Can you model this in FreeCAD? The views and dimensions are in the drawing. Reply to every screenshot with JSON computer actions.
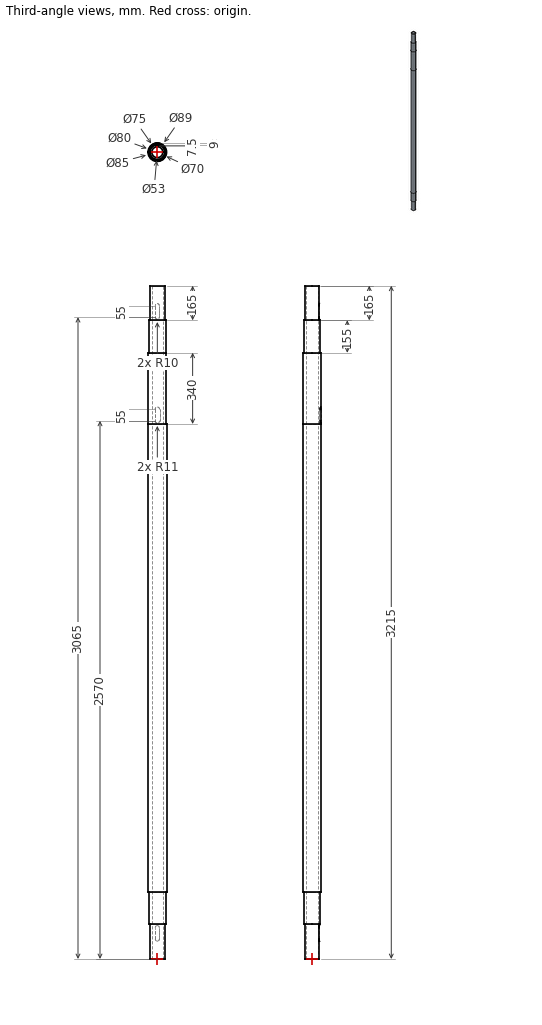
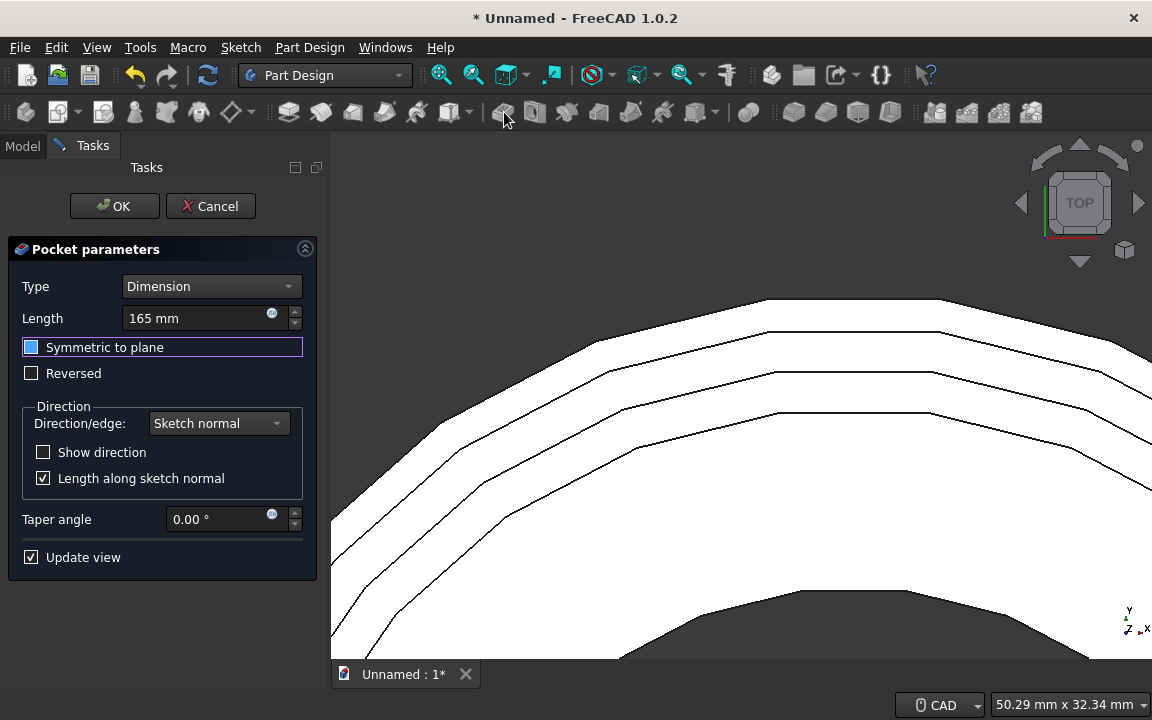
{"action": "left_click", "coordinate": [30, 373]}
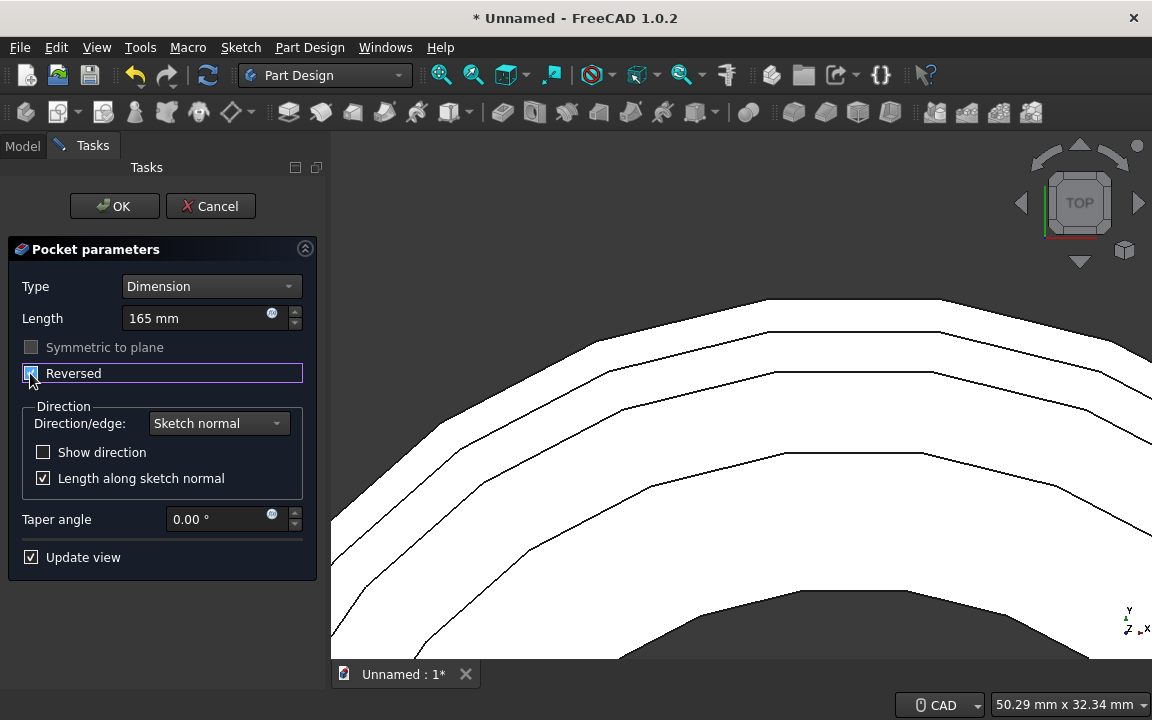
{"action": "left_click", "coordinate": [115, 206]}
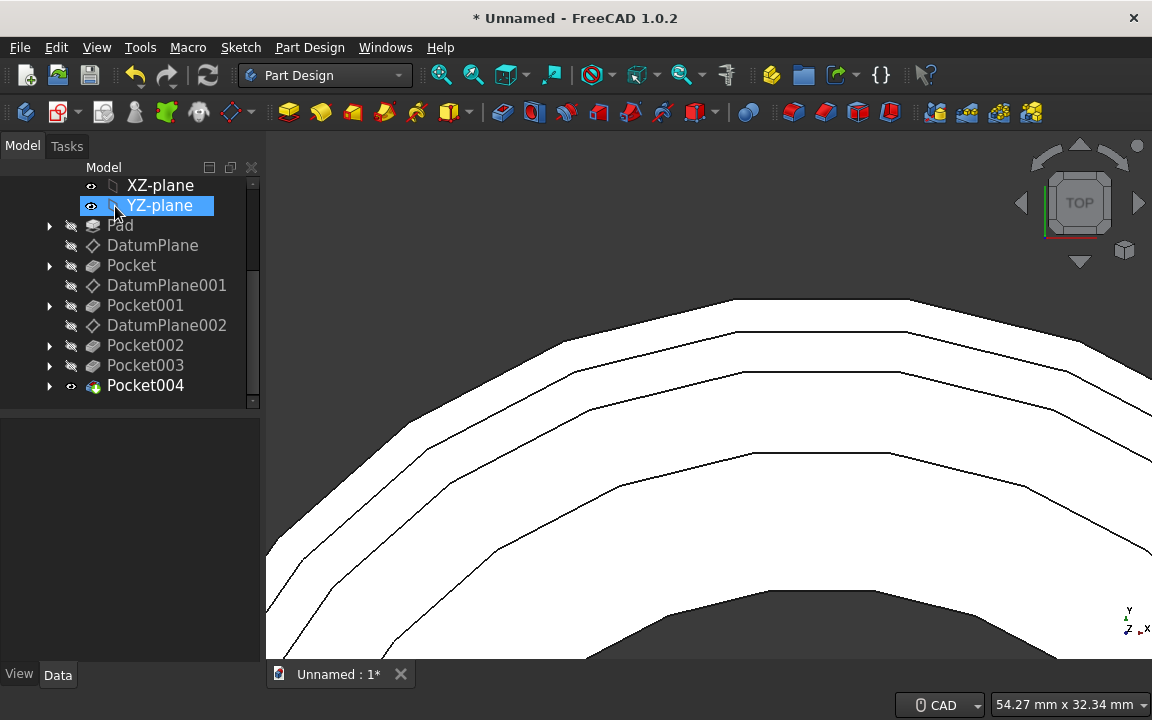
{"action": "left_click", "coordinate": [442, 76]}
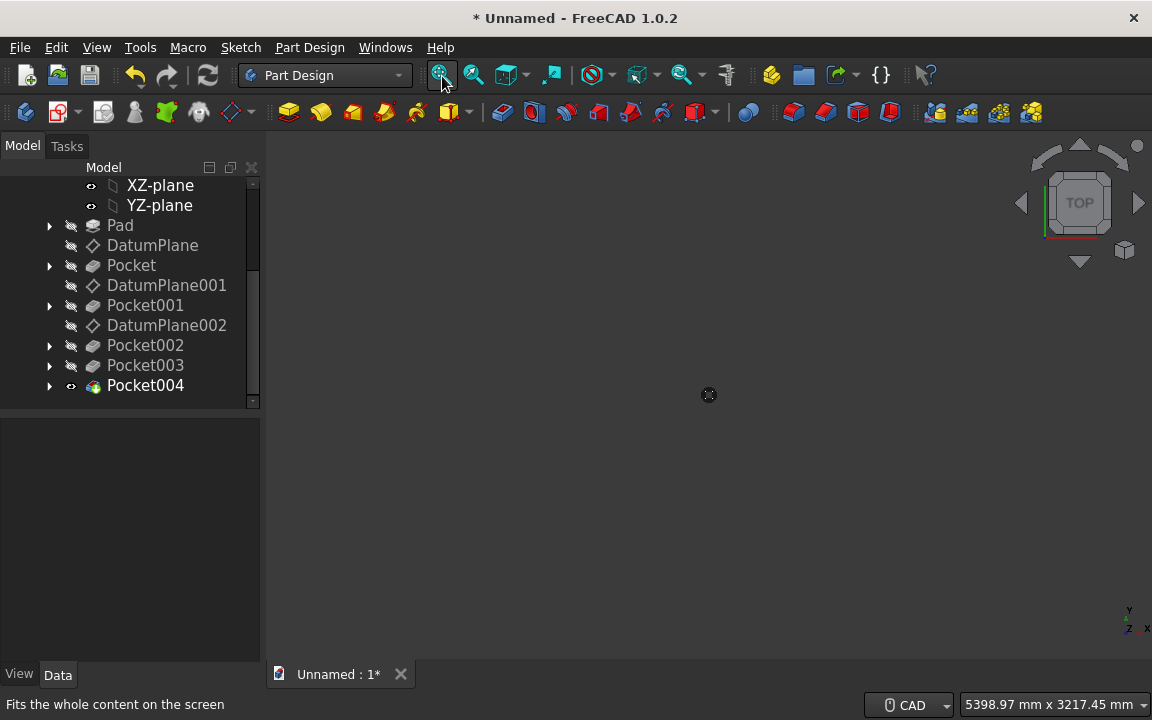
{"action": "scroll", "coordinate": [160, 281], "scroll_direction": "down", "scroll_amount": 3}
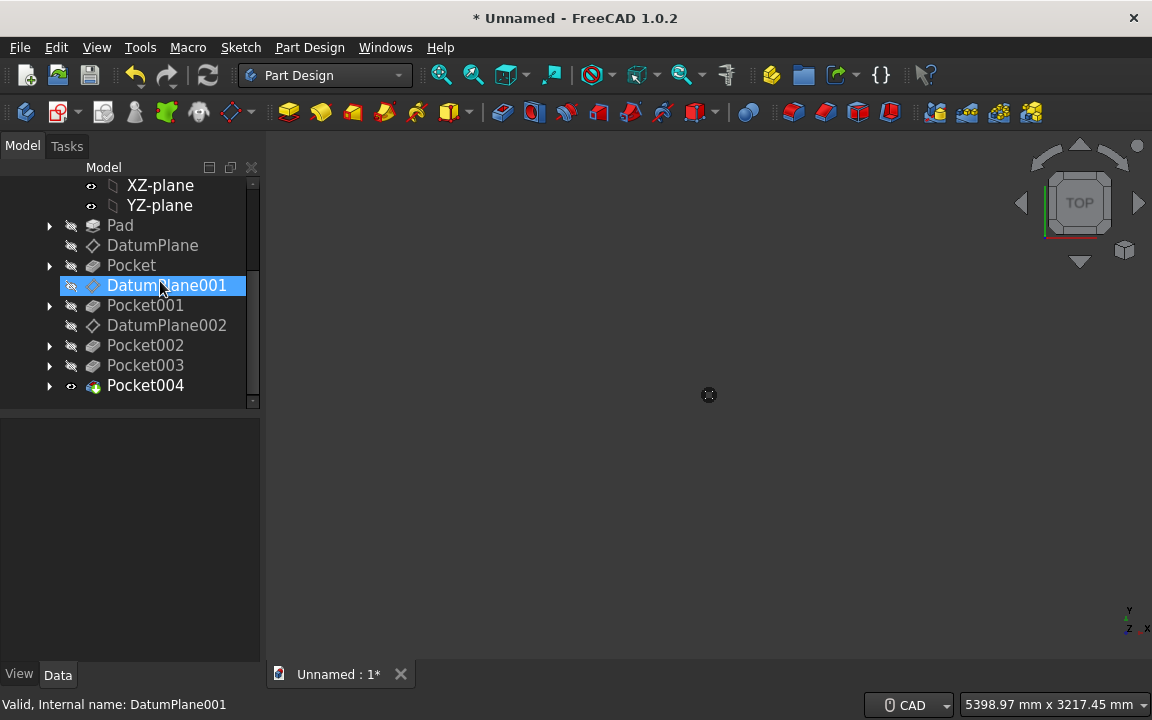
{"action": "scroll", "coordinate": [160, 281], "scroll_direction": "up", "scroll_amount": 15}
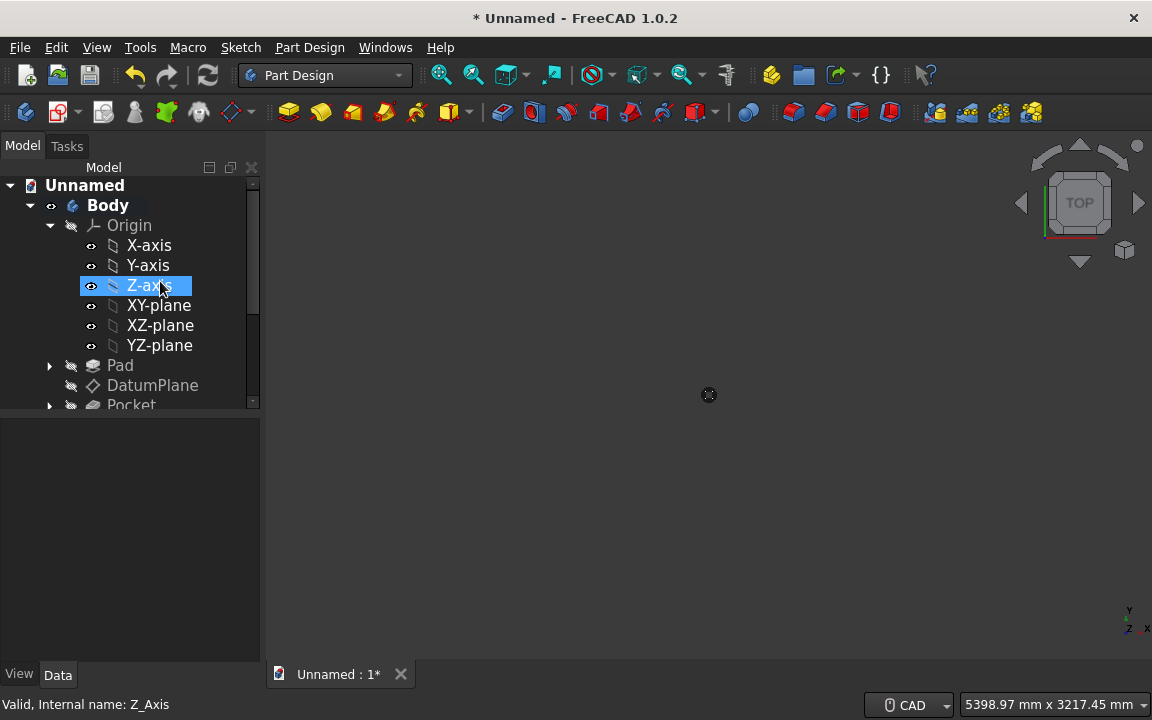
{"action": "left_click", "coordinate": [136, 306]}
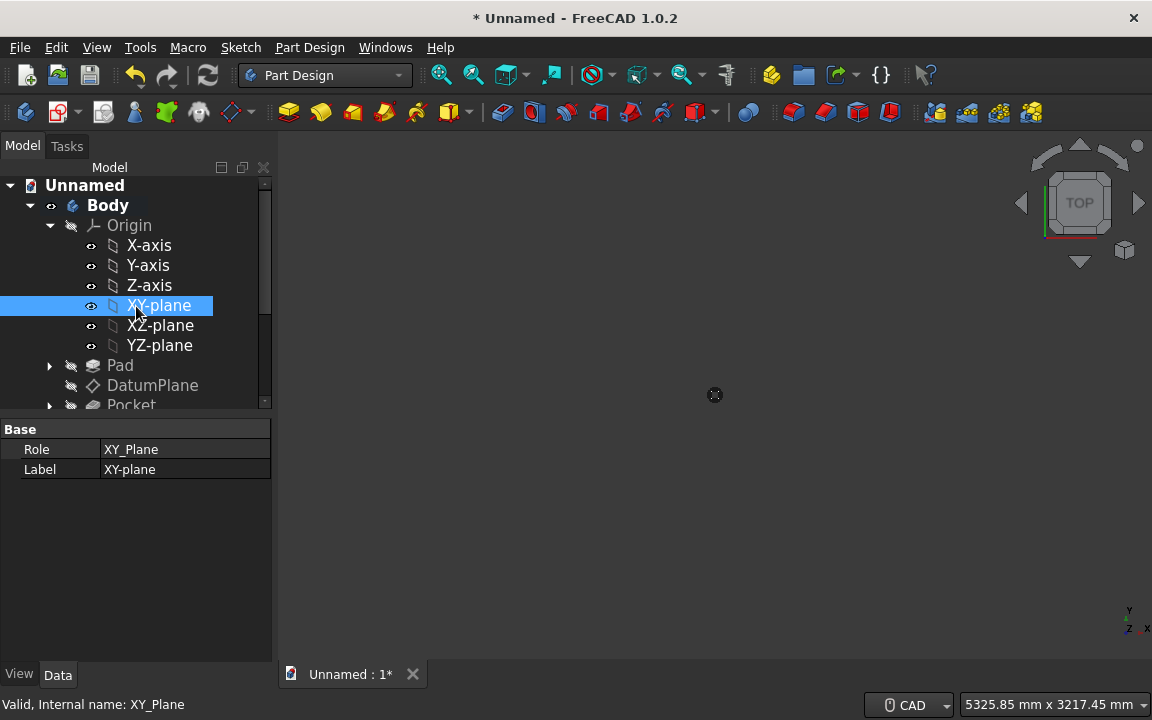
{"action": "left_click", "coordinate": [232, 112]}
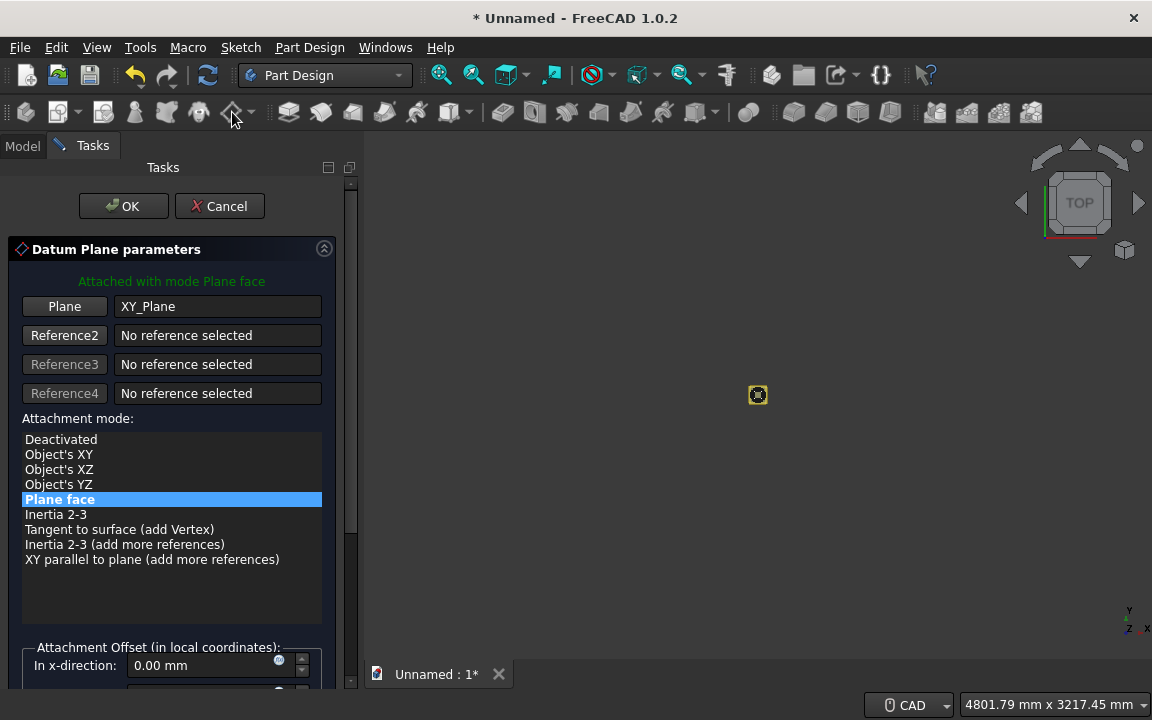
{"action": "scroll", "coordinate": [351, 432], "scroll_direction": "down", "scroll_amount": 2}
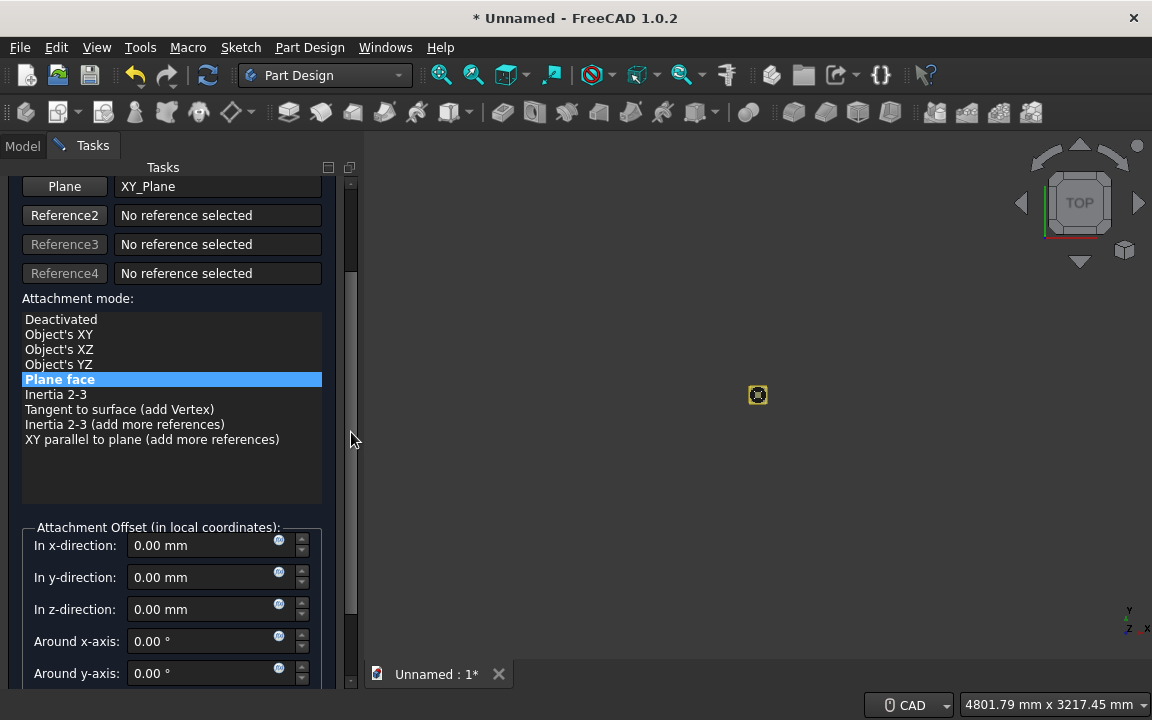
{"action": "triple_click", "coordinate": [210, 609]}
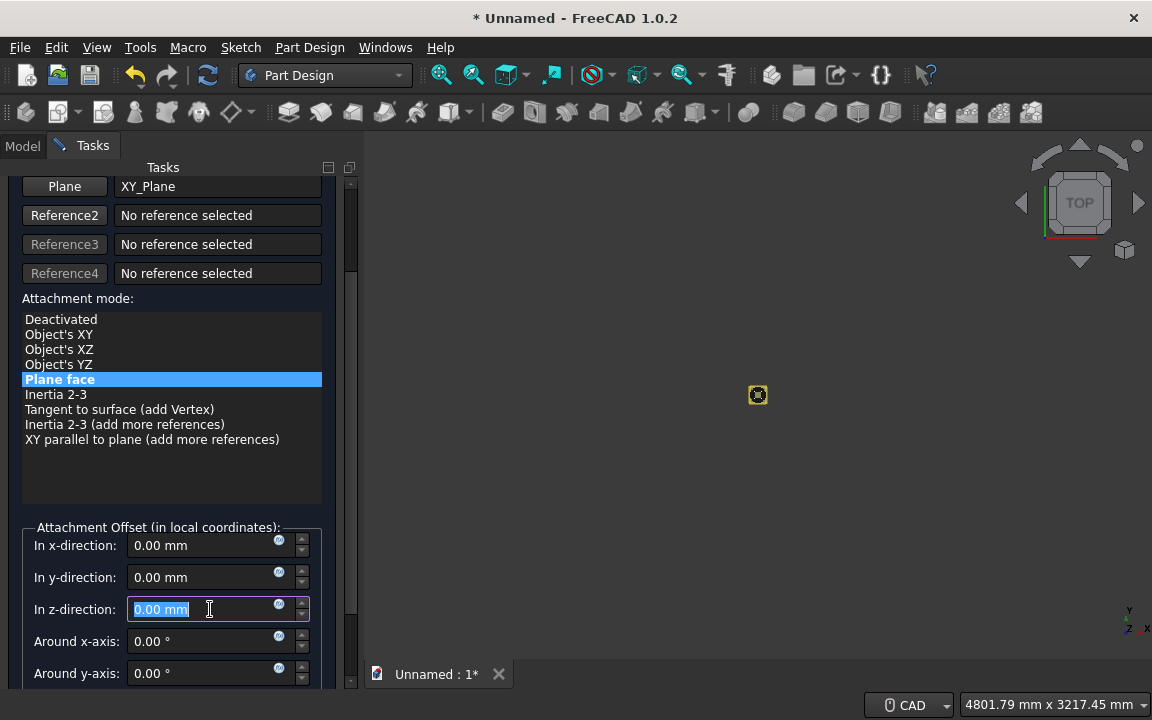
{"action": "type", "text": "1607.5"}
{"action": "key", "text": "Tab"}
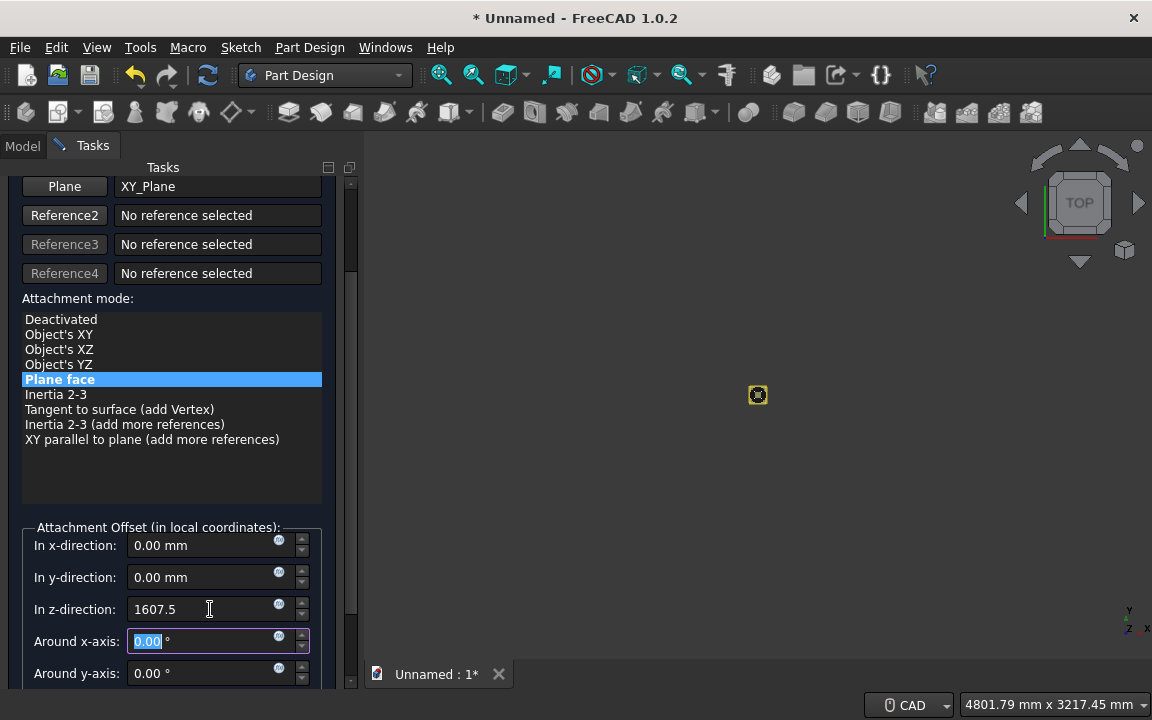
{"action": "scroll", "coordinate": [351, 432], "scroll_direction": "up", "scroll_amount": 3}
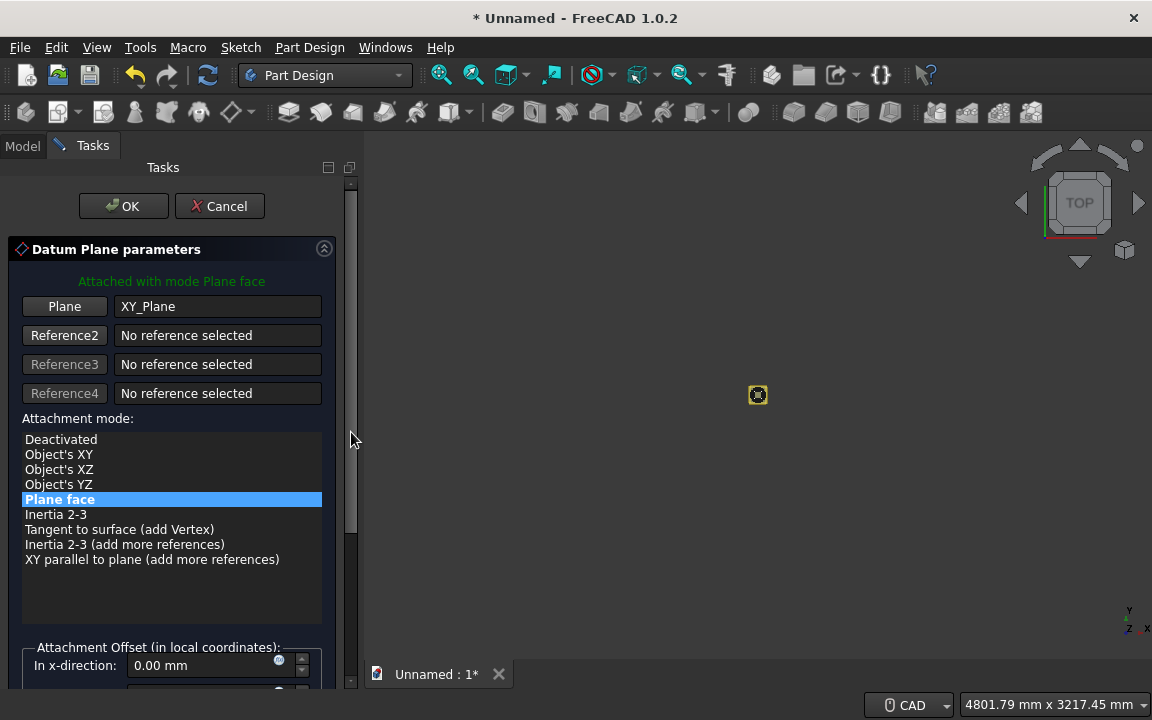
{"action": "left_click", "coordinate": [124, 206]}